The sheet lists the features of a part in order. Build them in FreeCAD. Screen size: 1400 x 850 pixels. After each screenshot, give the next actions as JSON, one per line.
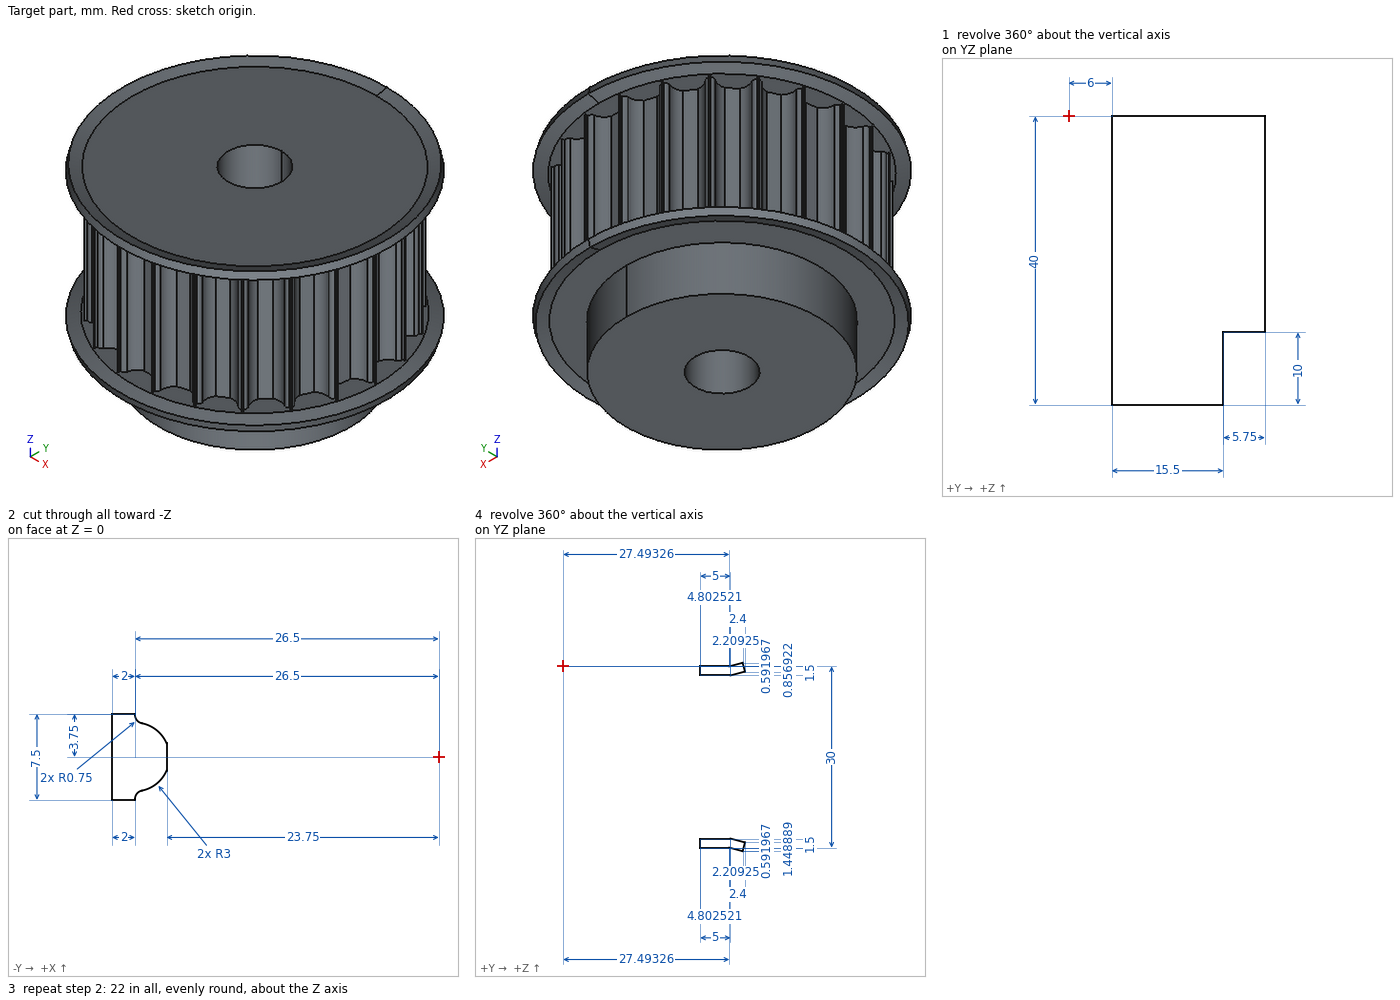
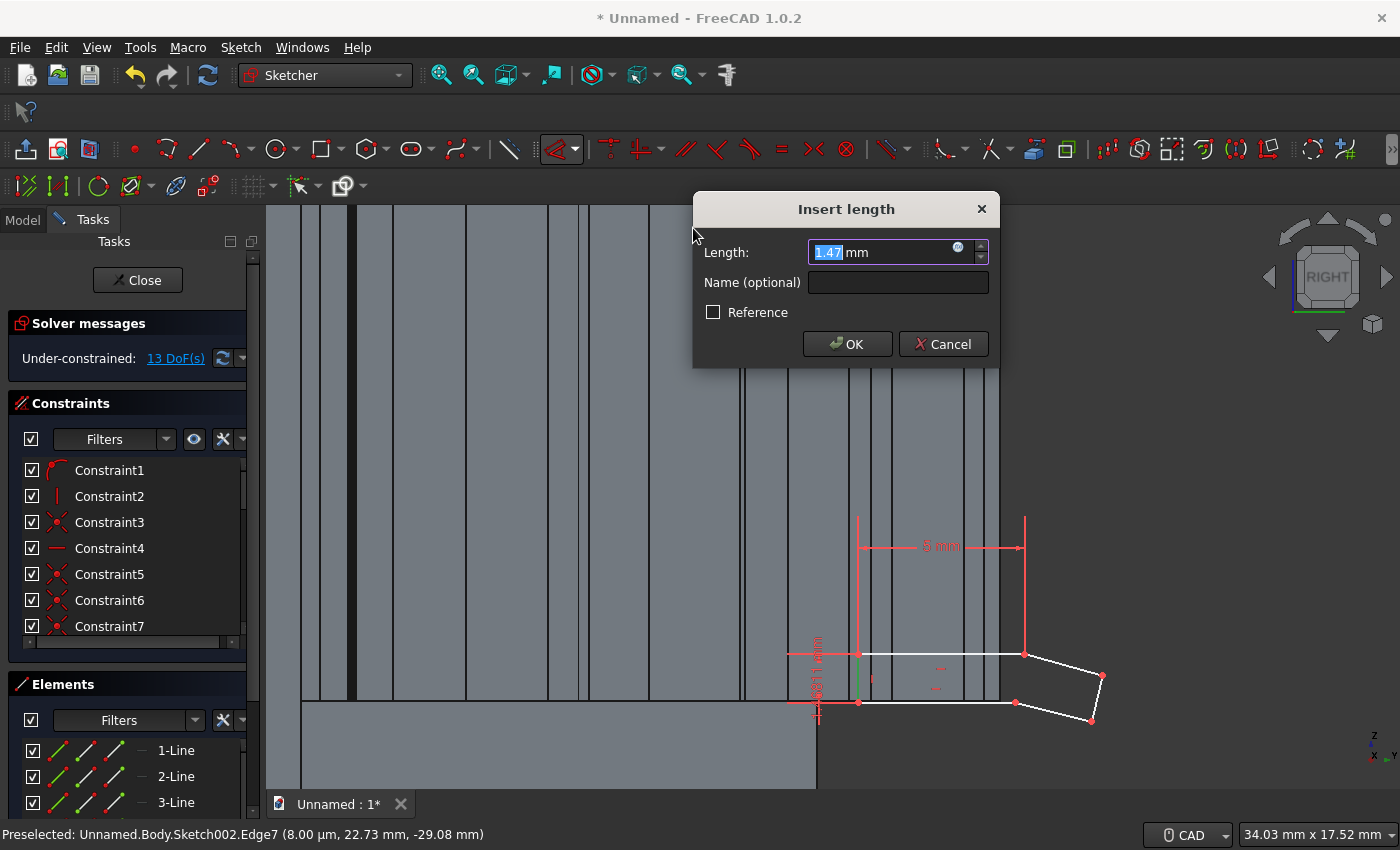
{"action": "type", "text": "1.5"}
{"action": "key", "text": "Return"}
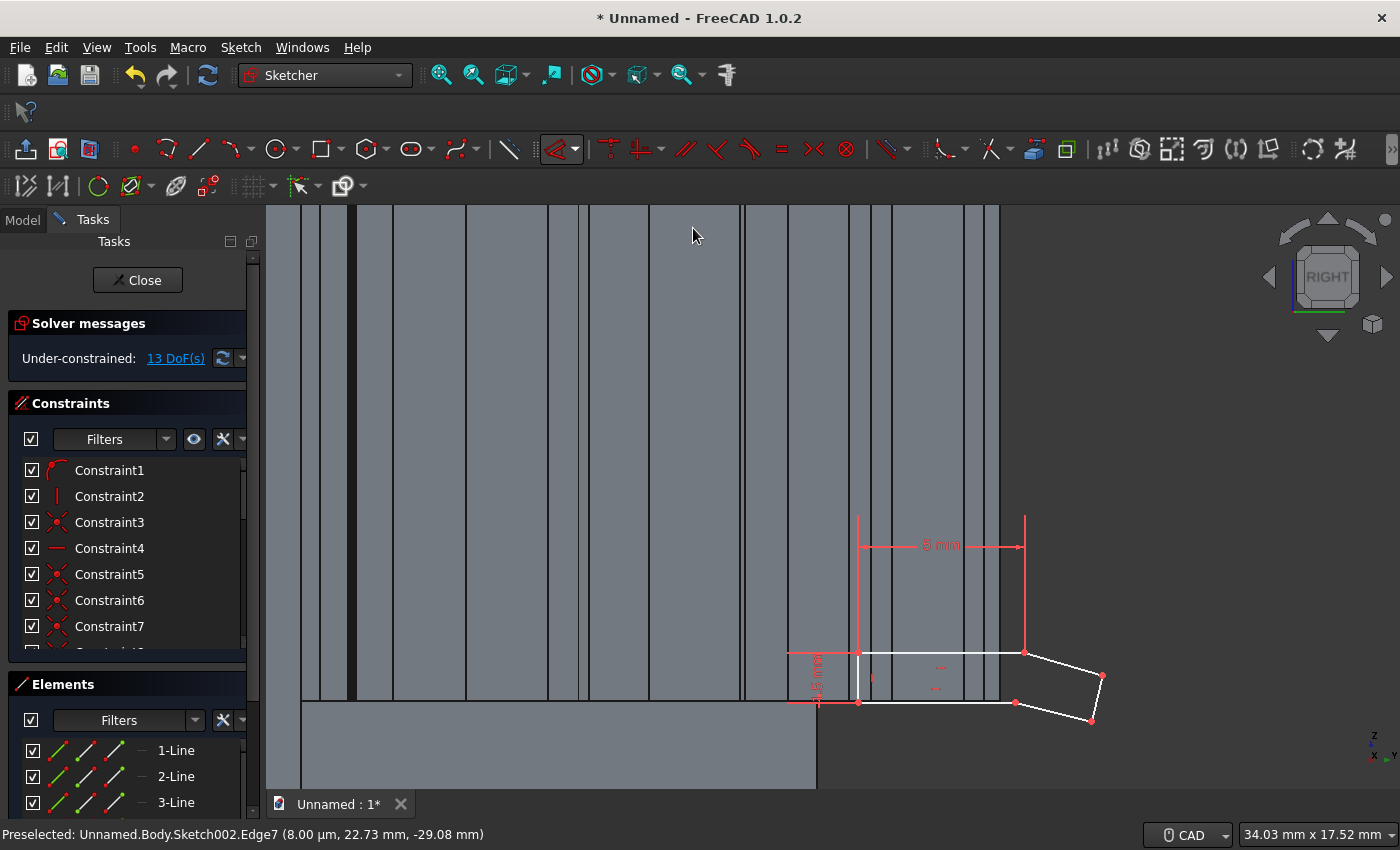
{"action": "left_click", "coordinate": [858, 703]}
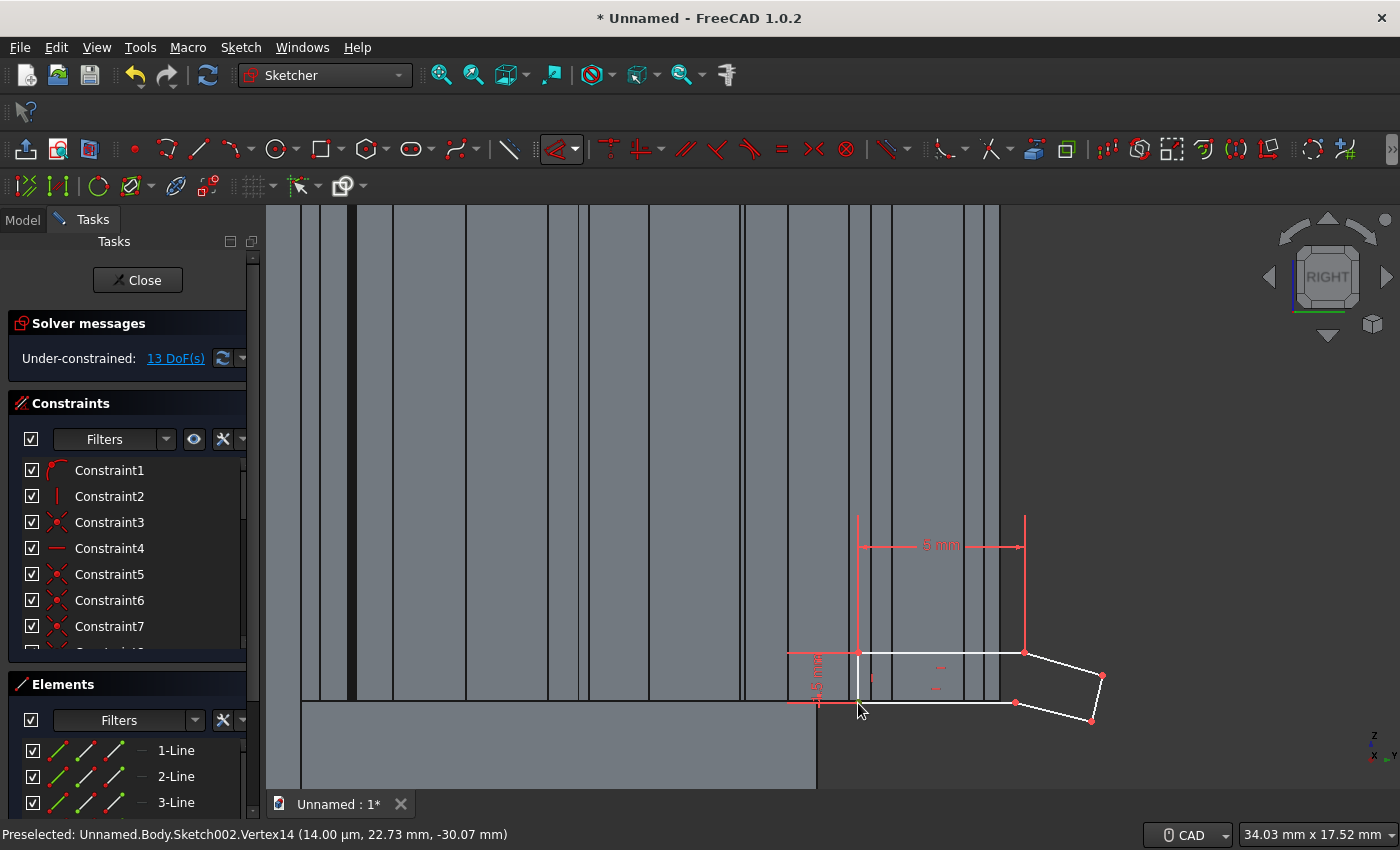
{"action": "key", "text": "i"}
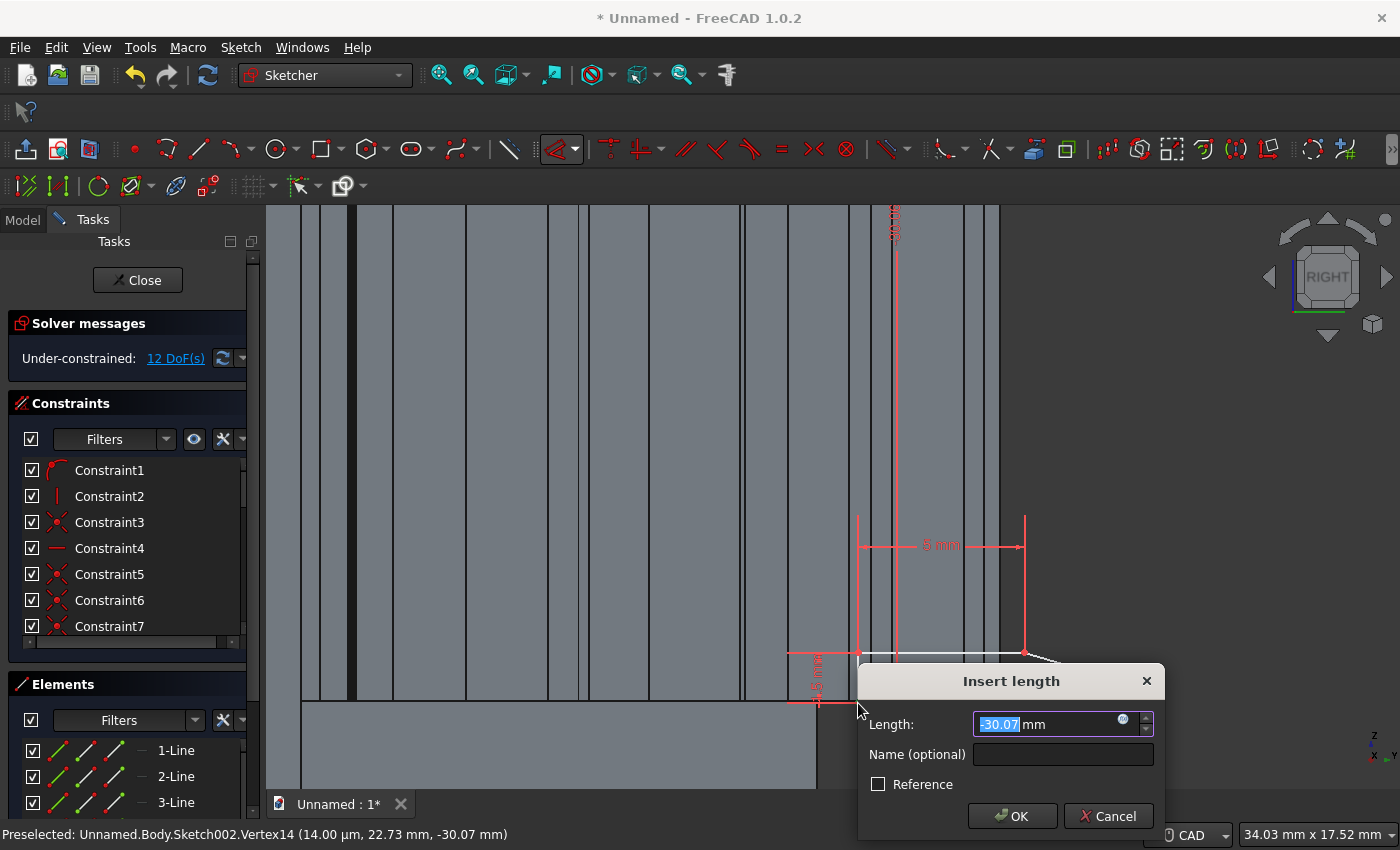
{"action": "type", "text": "-30"}
{"action": "key", "text": "Return"}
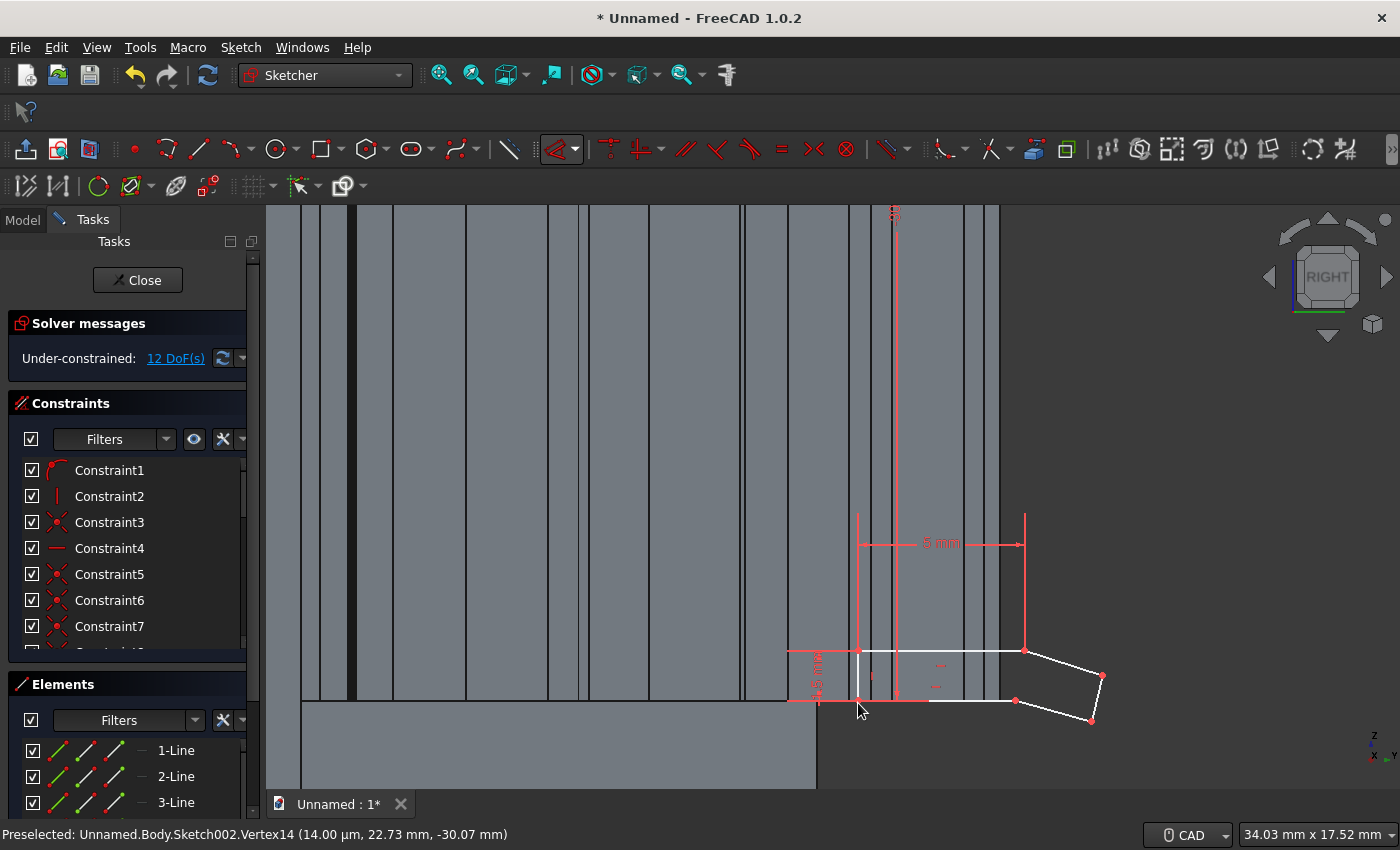
{"action": "scroll", "coordinate": [859, 669], "scroll_direction": "down", "scroll_amount": 5}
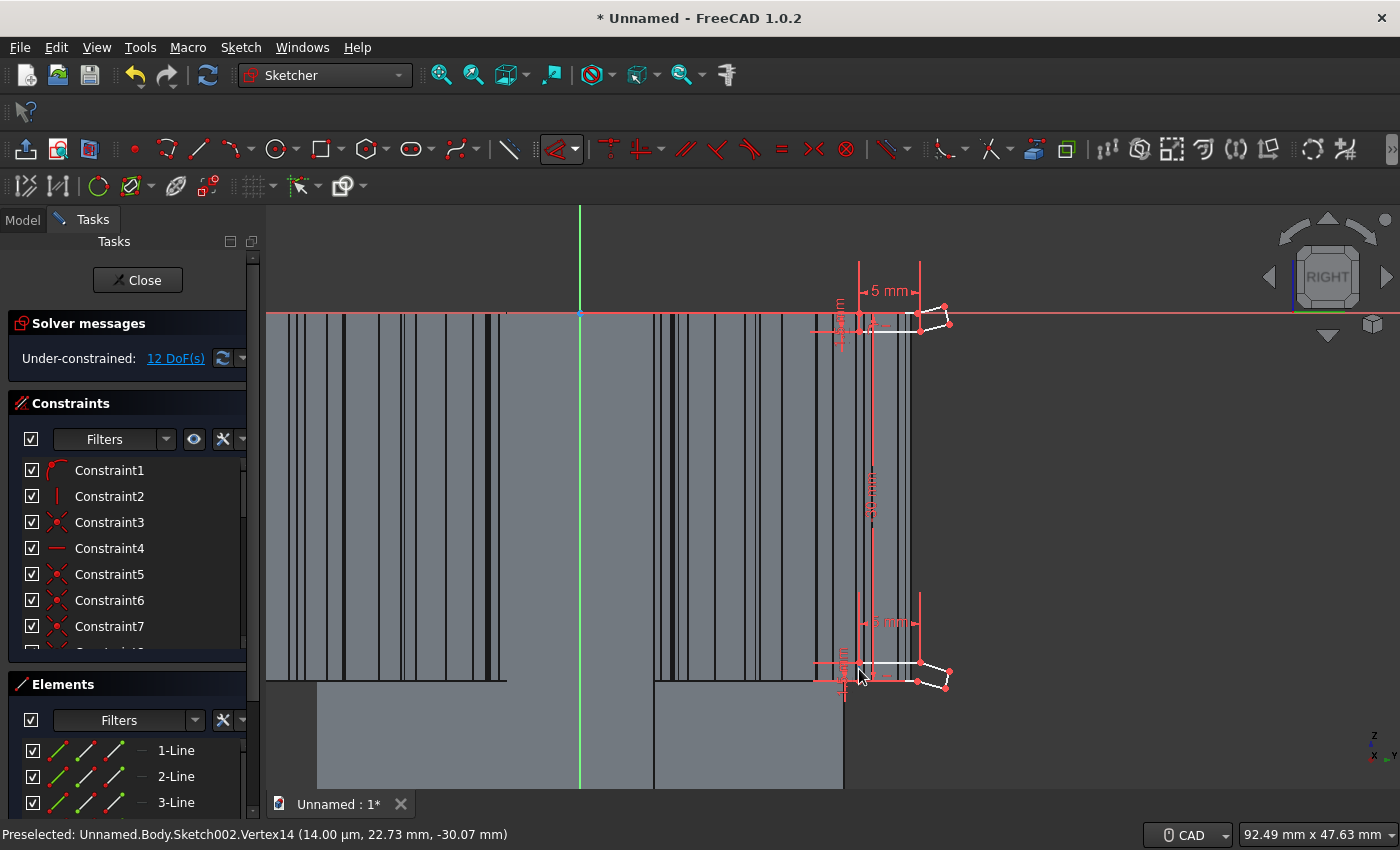
{"action": "scroll", "coordinate": [929, 330], "scroll_direction": "up", "scroll_amount": 3}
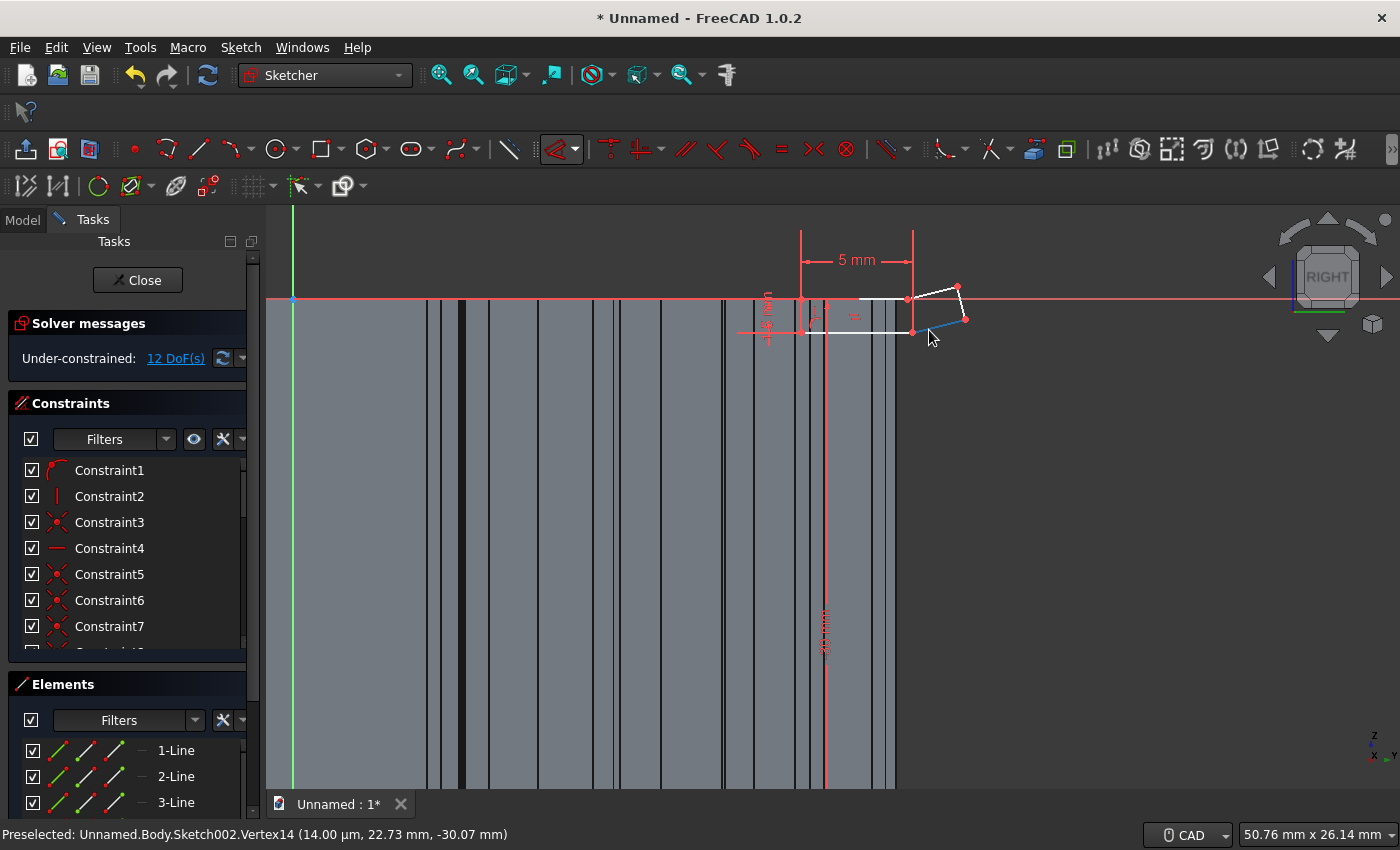
{"action": "left_click", "coordinate": [928, 329]}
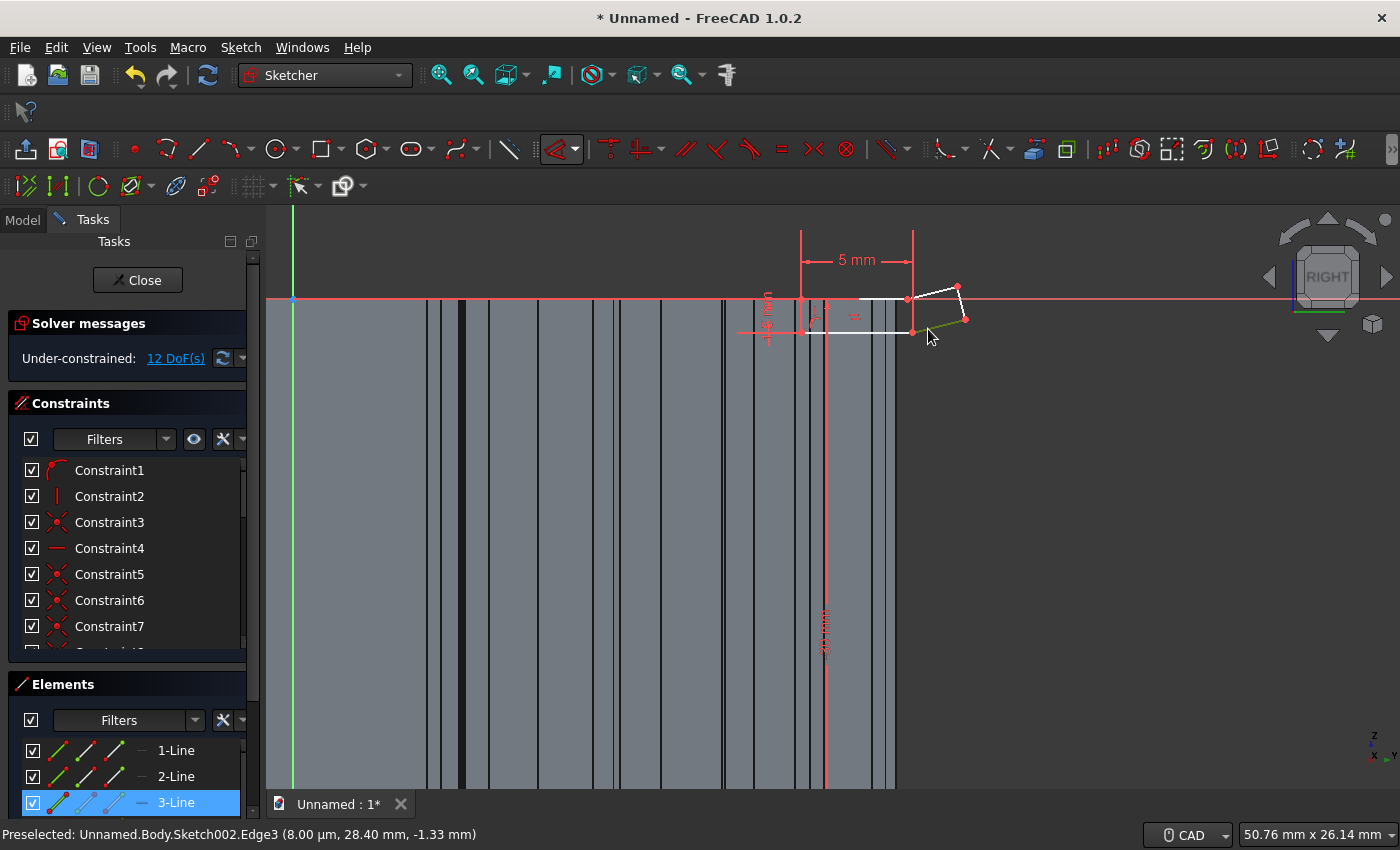
{"action": "left_click", "coordinate": [578, 150]}